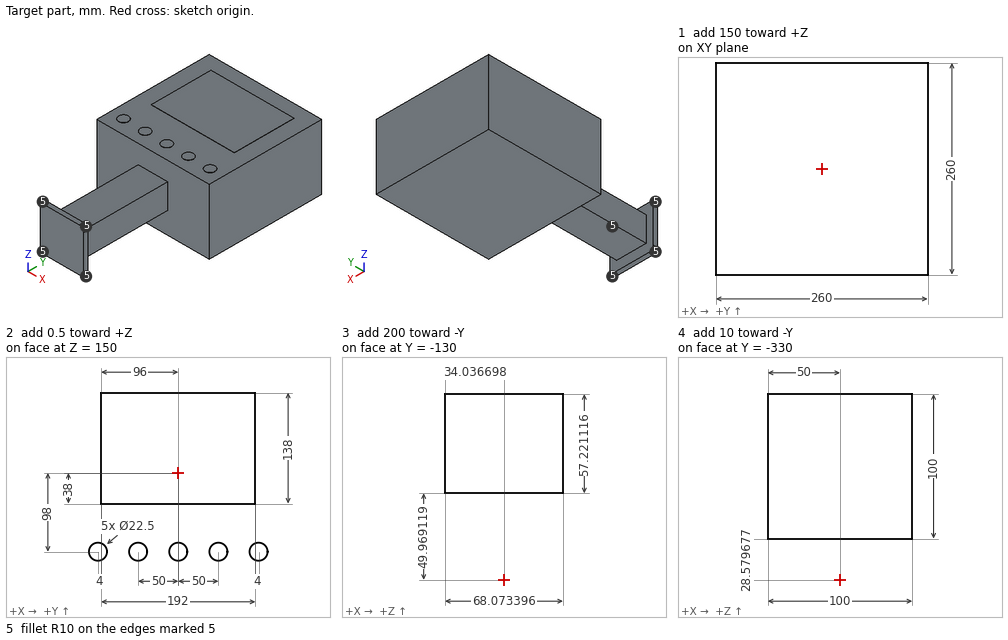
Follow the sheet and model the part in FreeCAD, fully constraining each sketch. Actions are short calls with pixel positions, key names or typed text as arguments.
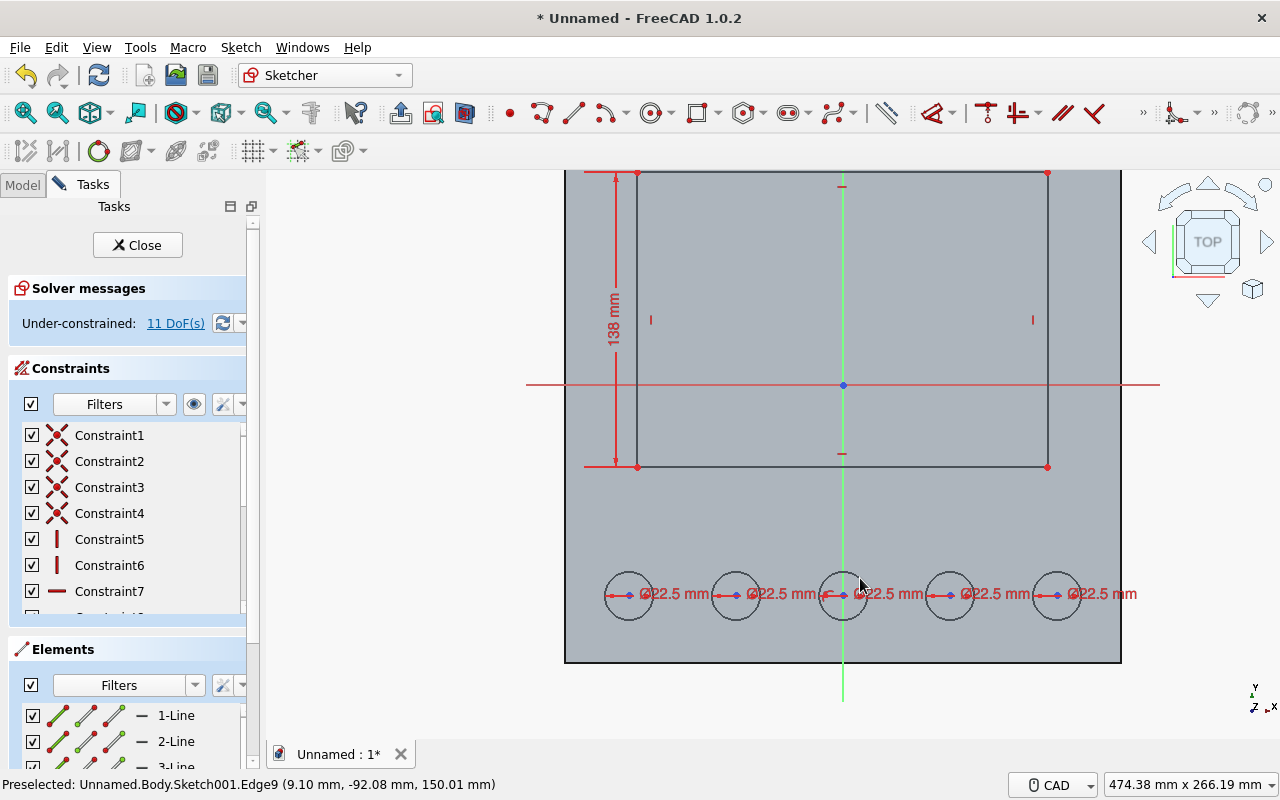
click(629, 596)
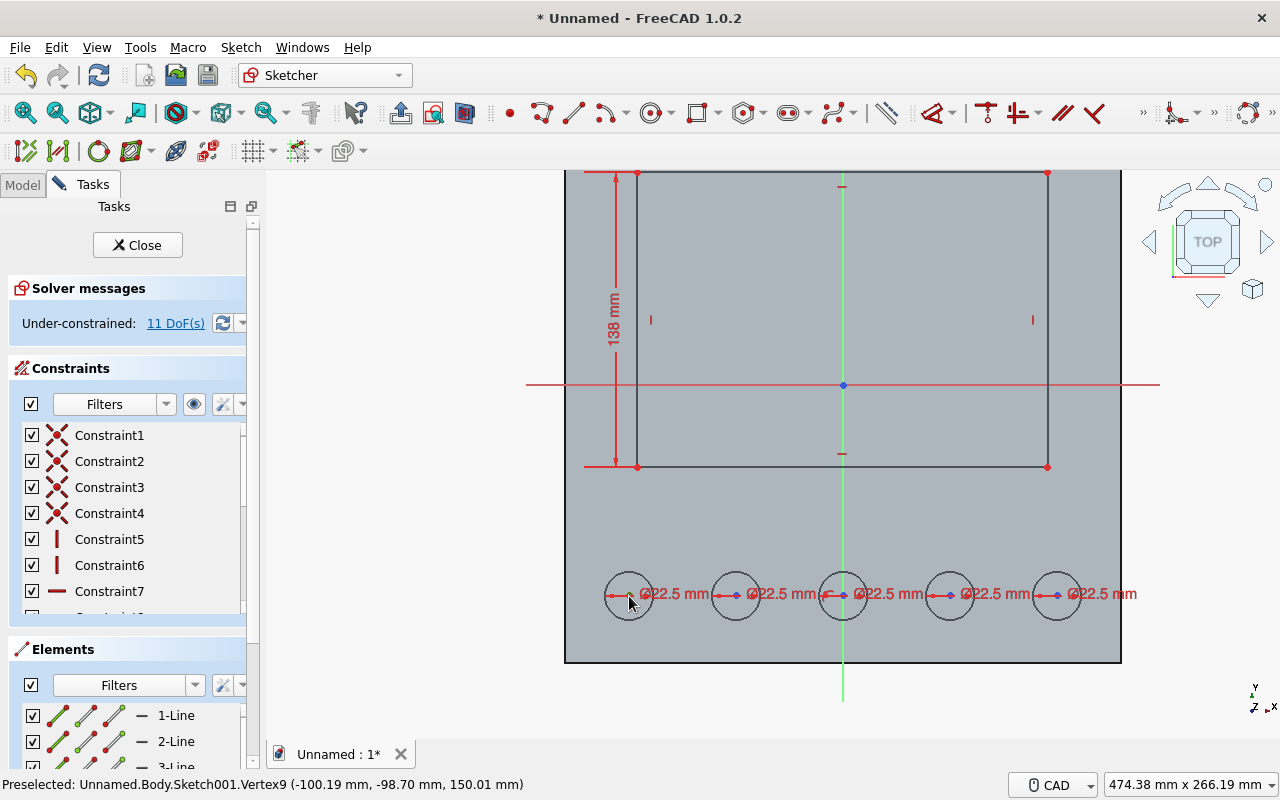
click(736, 596)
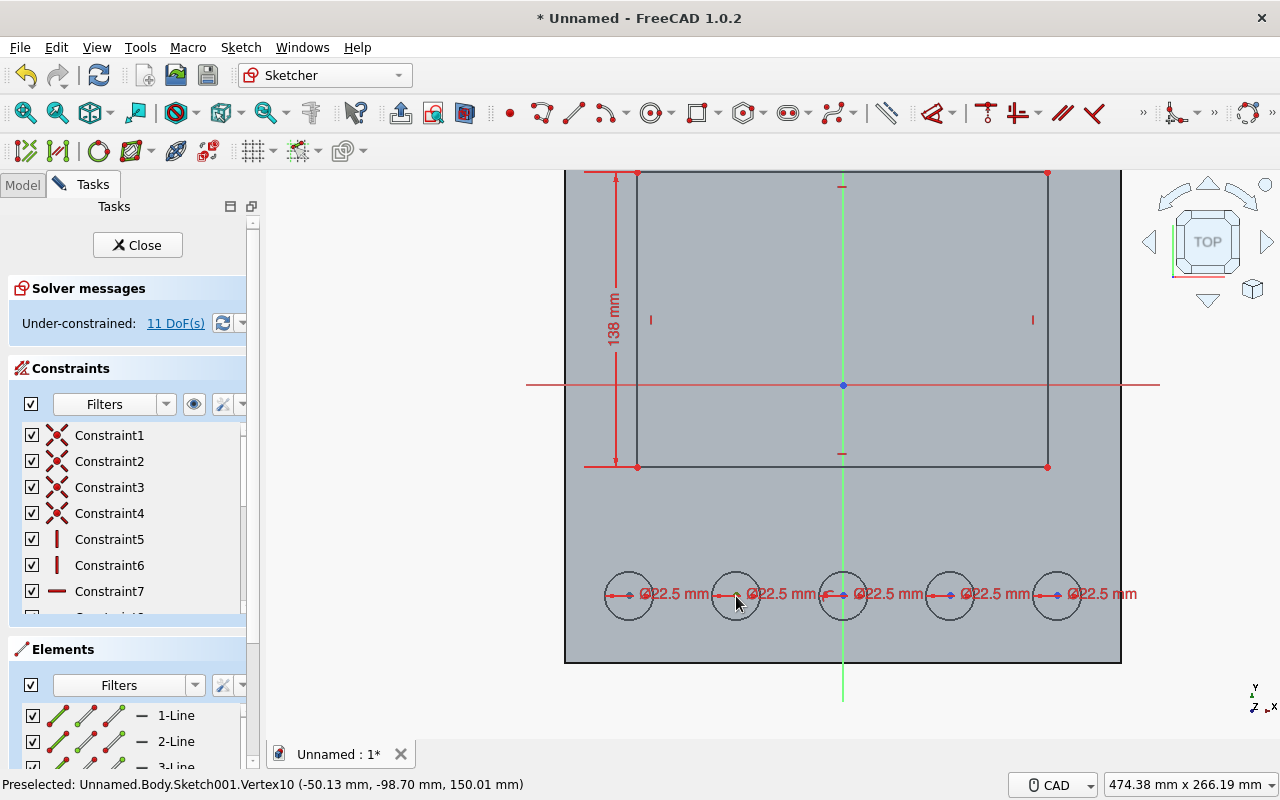
key(h)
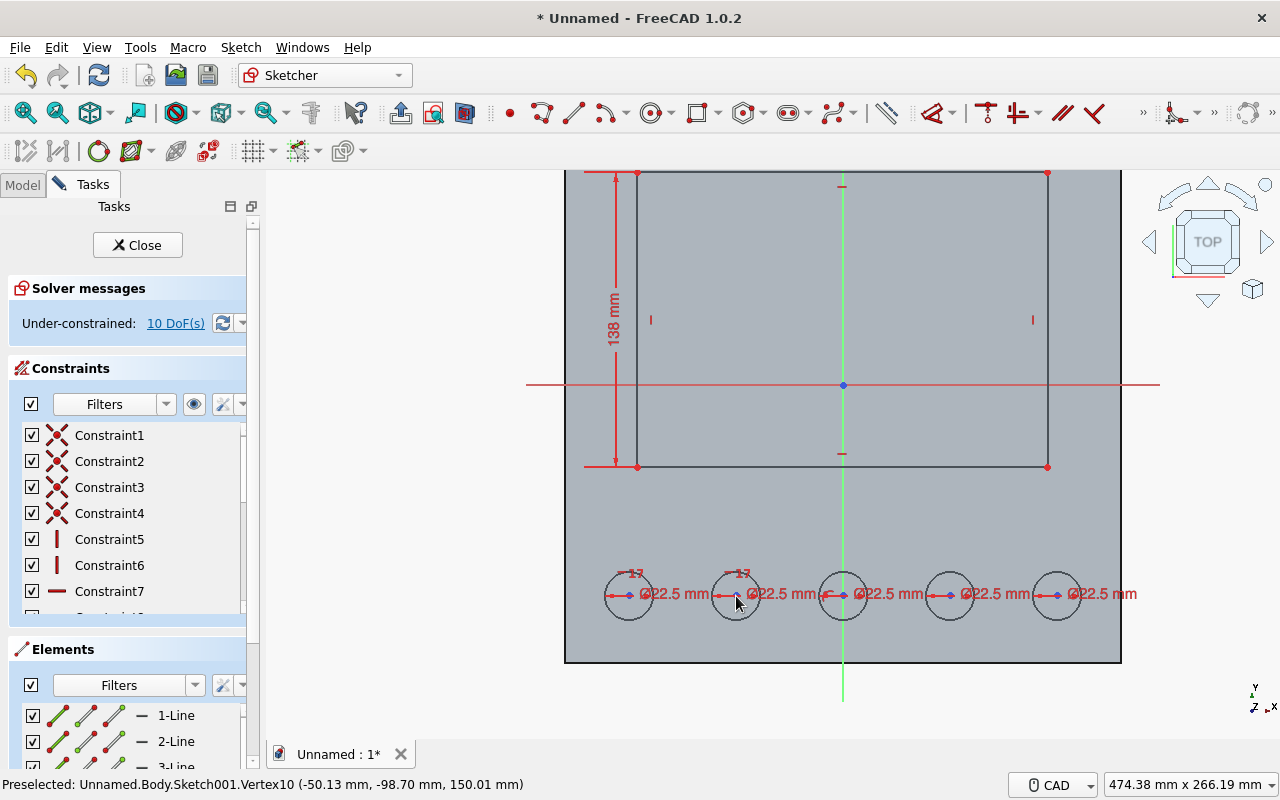
click(736, 596)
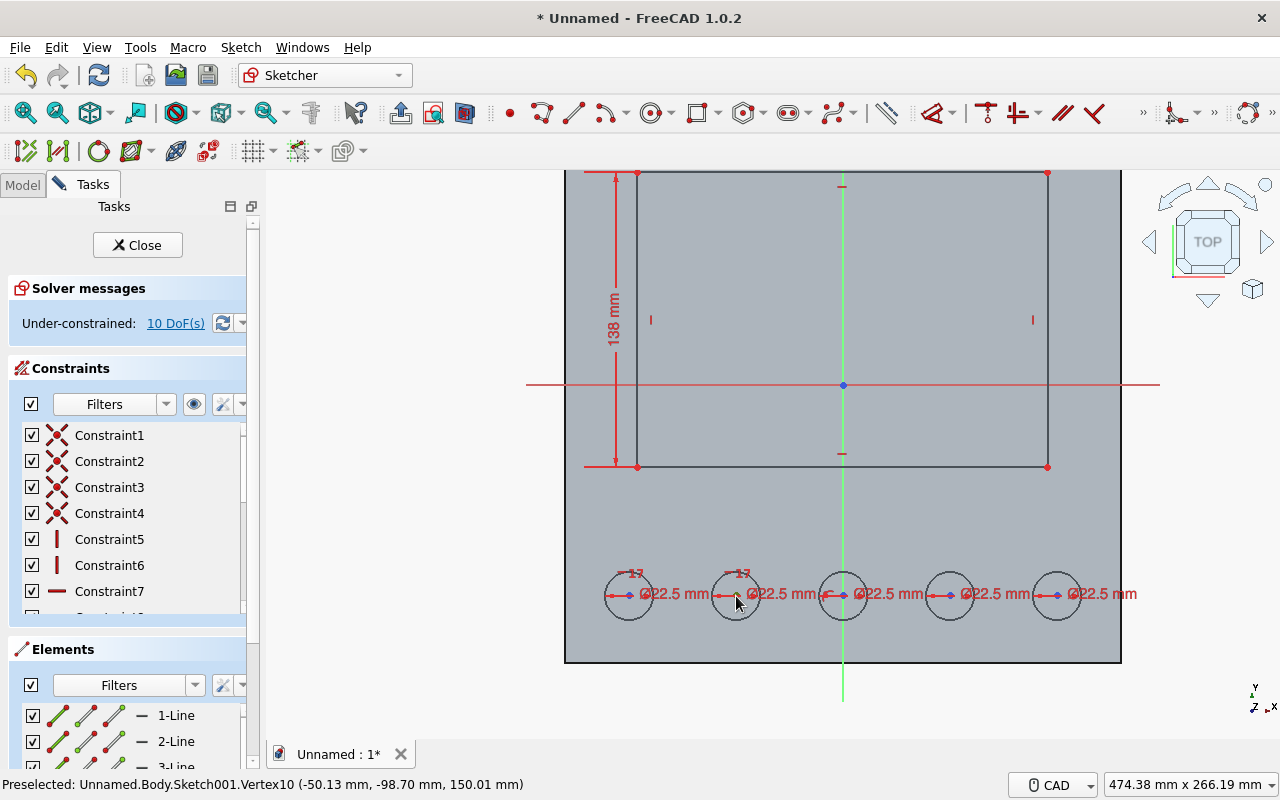
click(950, 596)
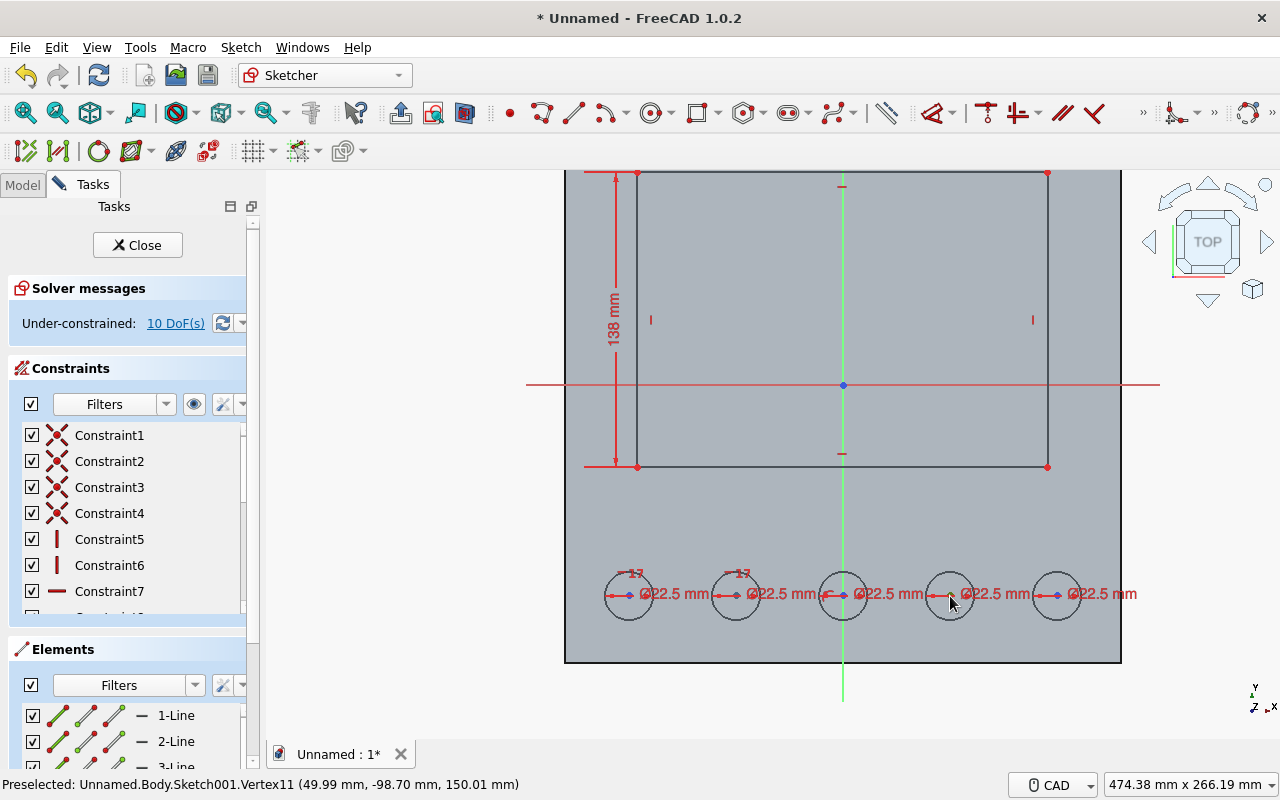
key(h)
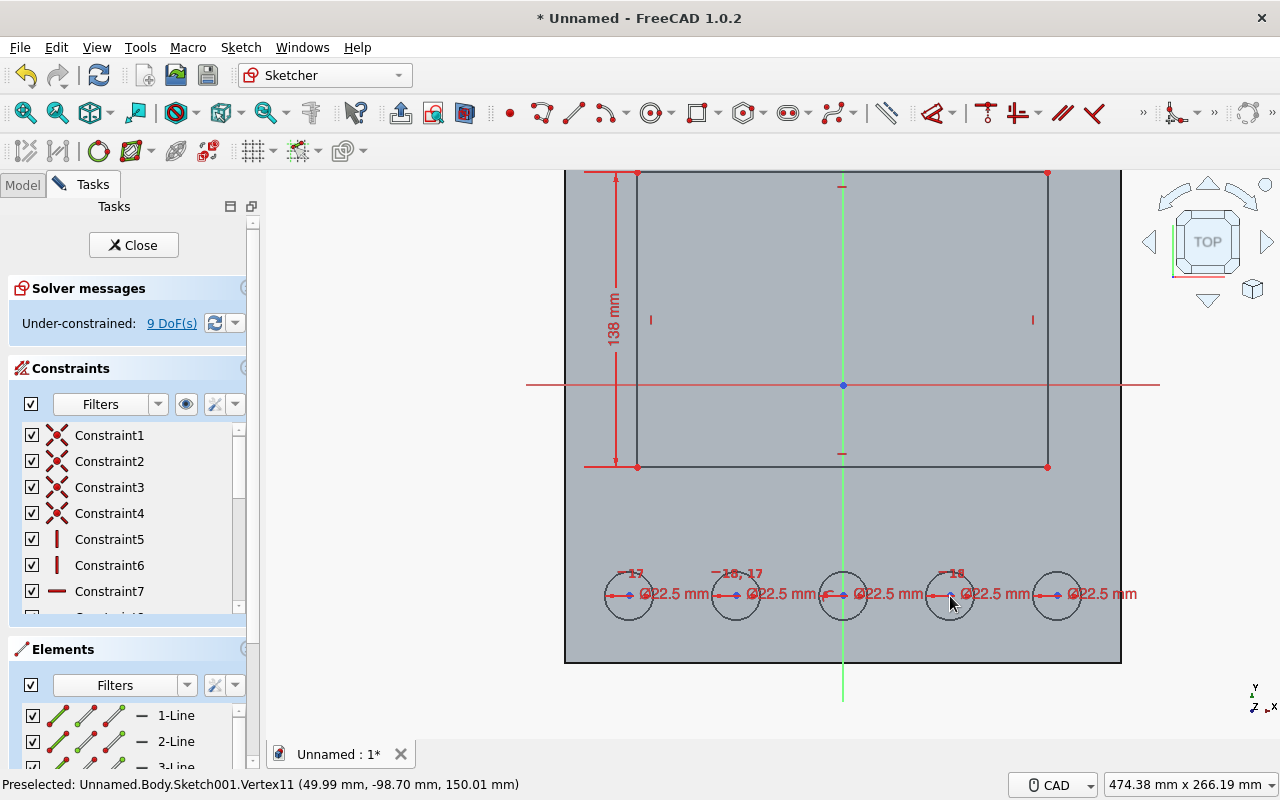
click(950, 596)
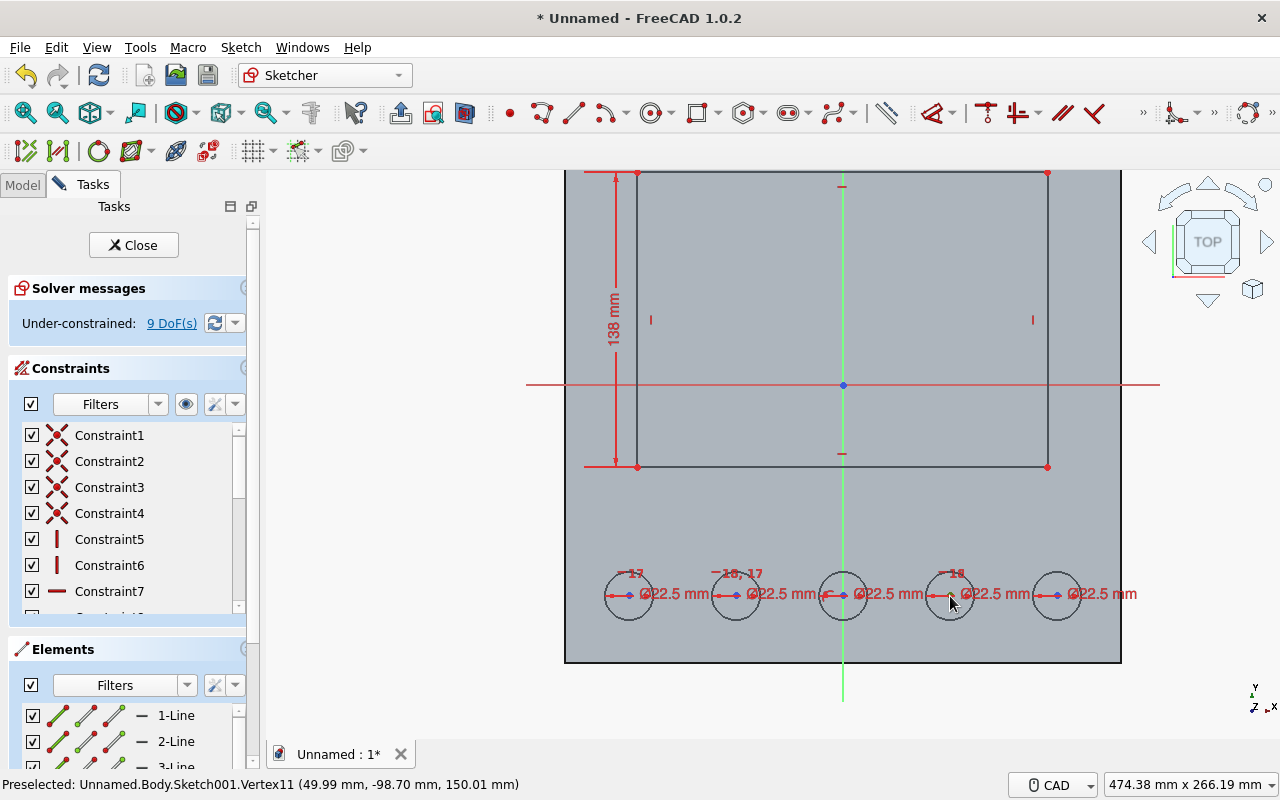
click(1057, 596)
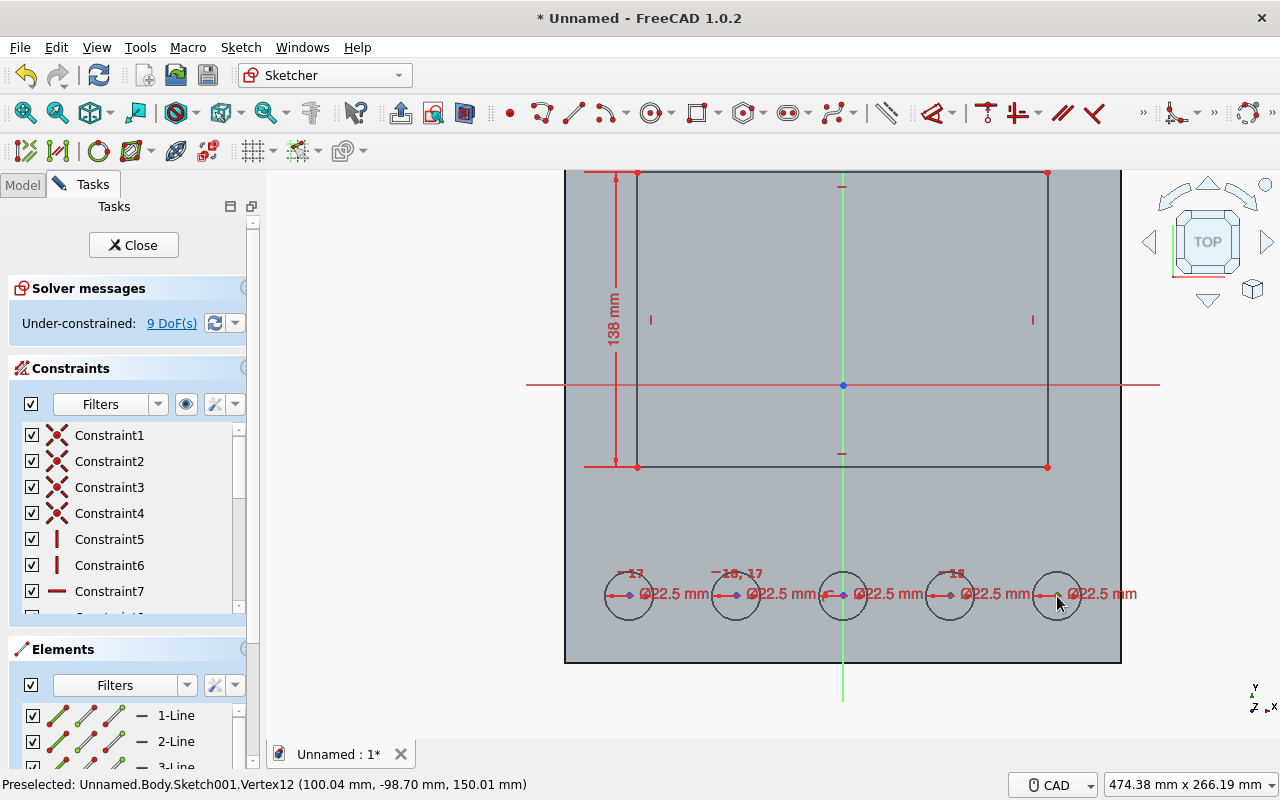
key(h)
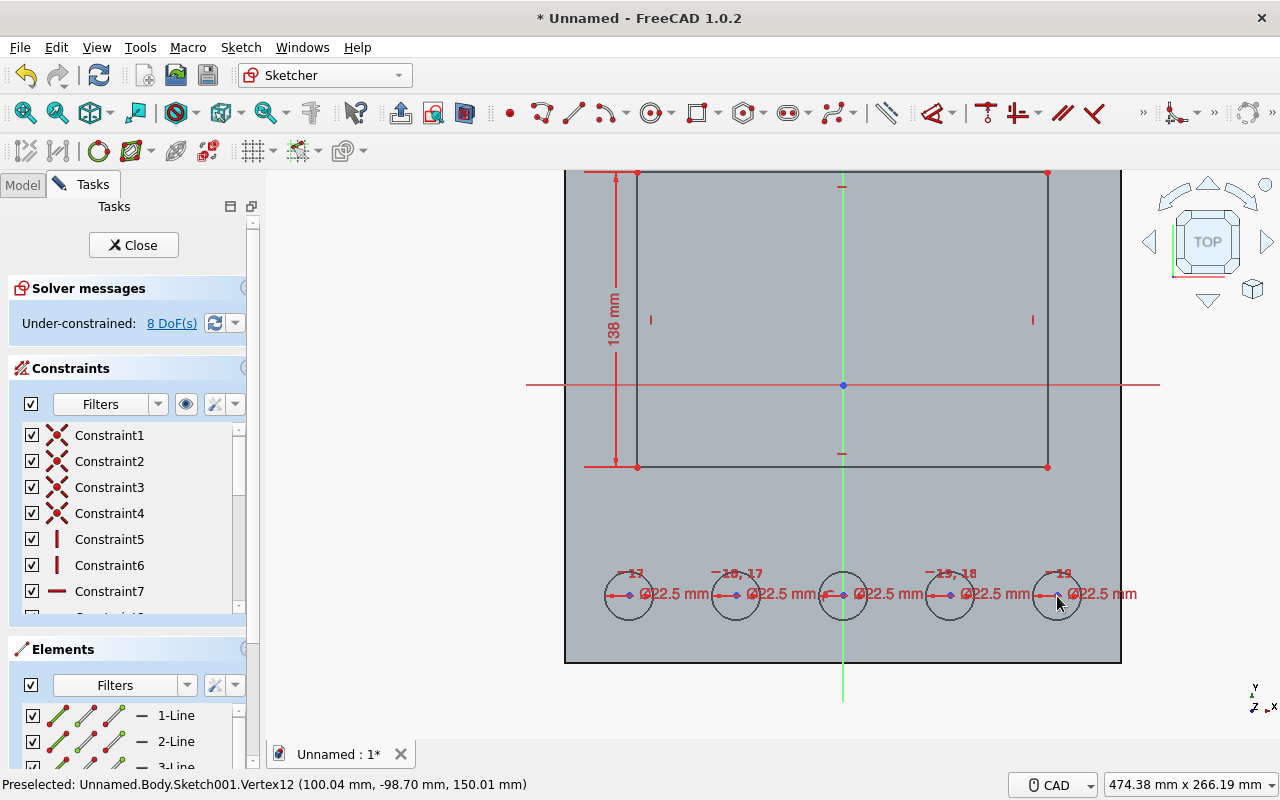
click(736, 596)